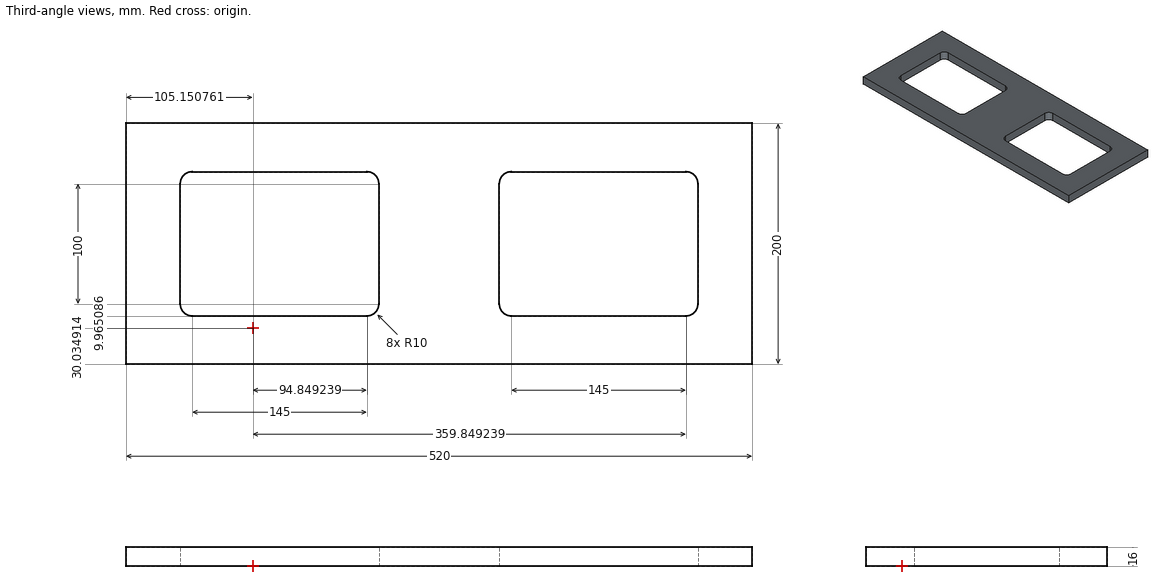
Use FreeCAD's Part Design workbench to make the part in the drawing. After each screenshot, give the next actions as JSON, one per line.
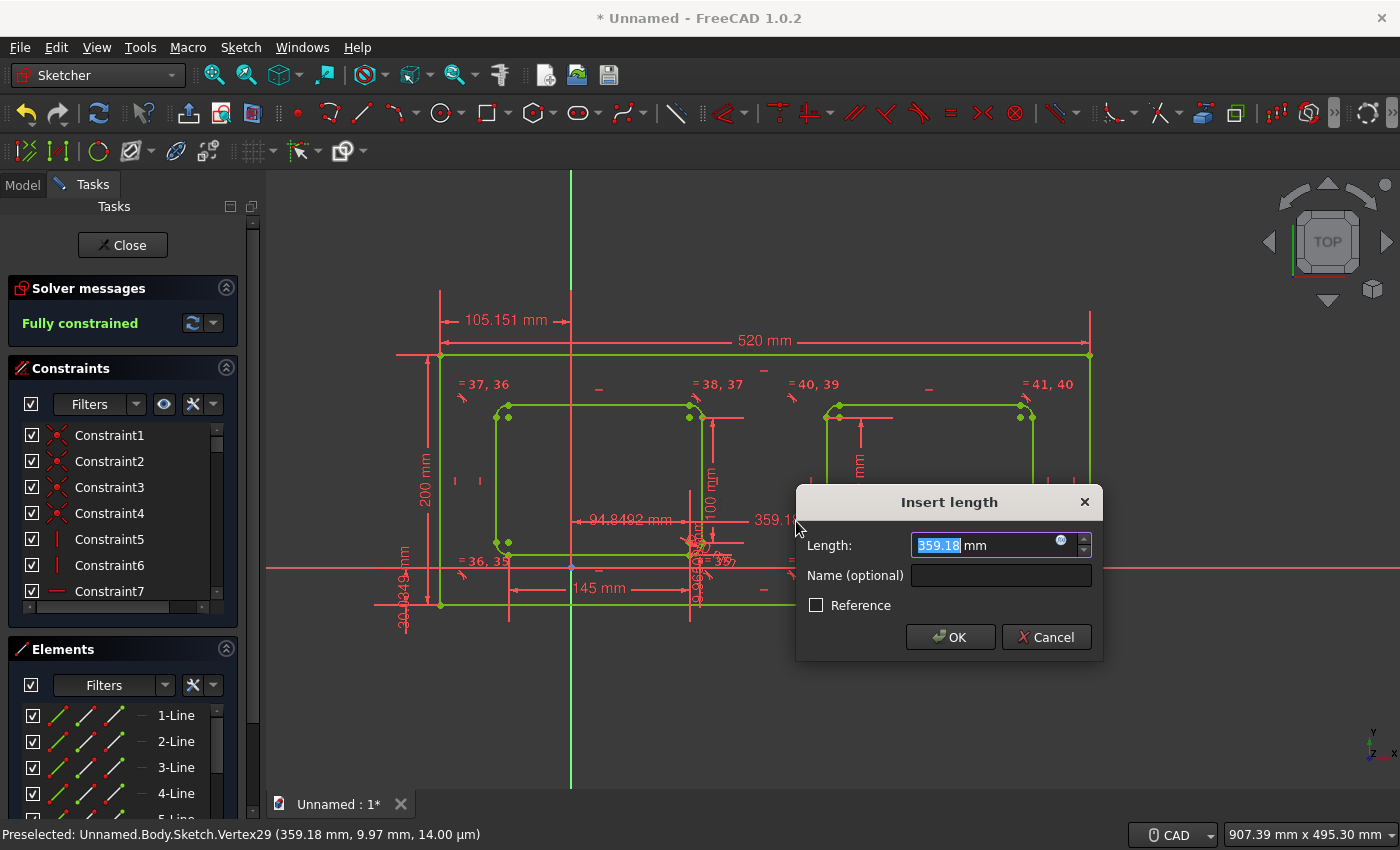
{"action": "type", "text": "359.849239"}
{"action": "key", "text": "Return"}
{"action": "key", "text": "Escape"}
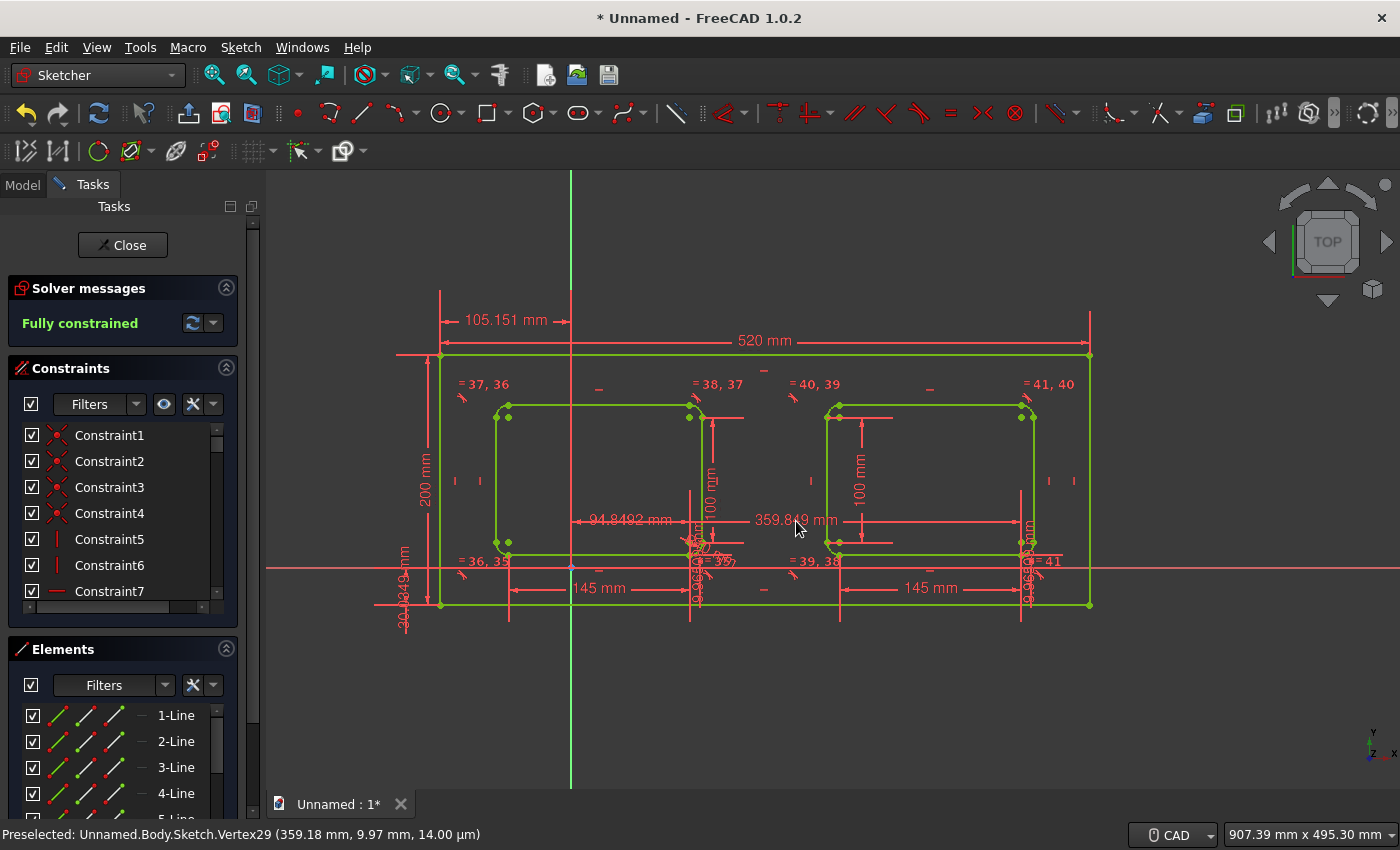
{"action": "left_click", "coordinate": [123, 245]}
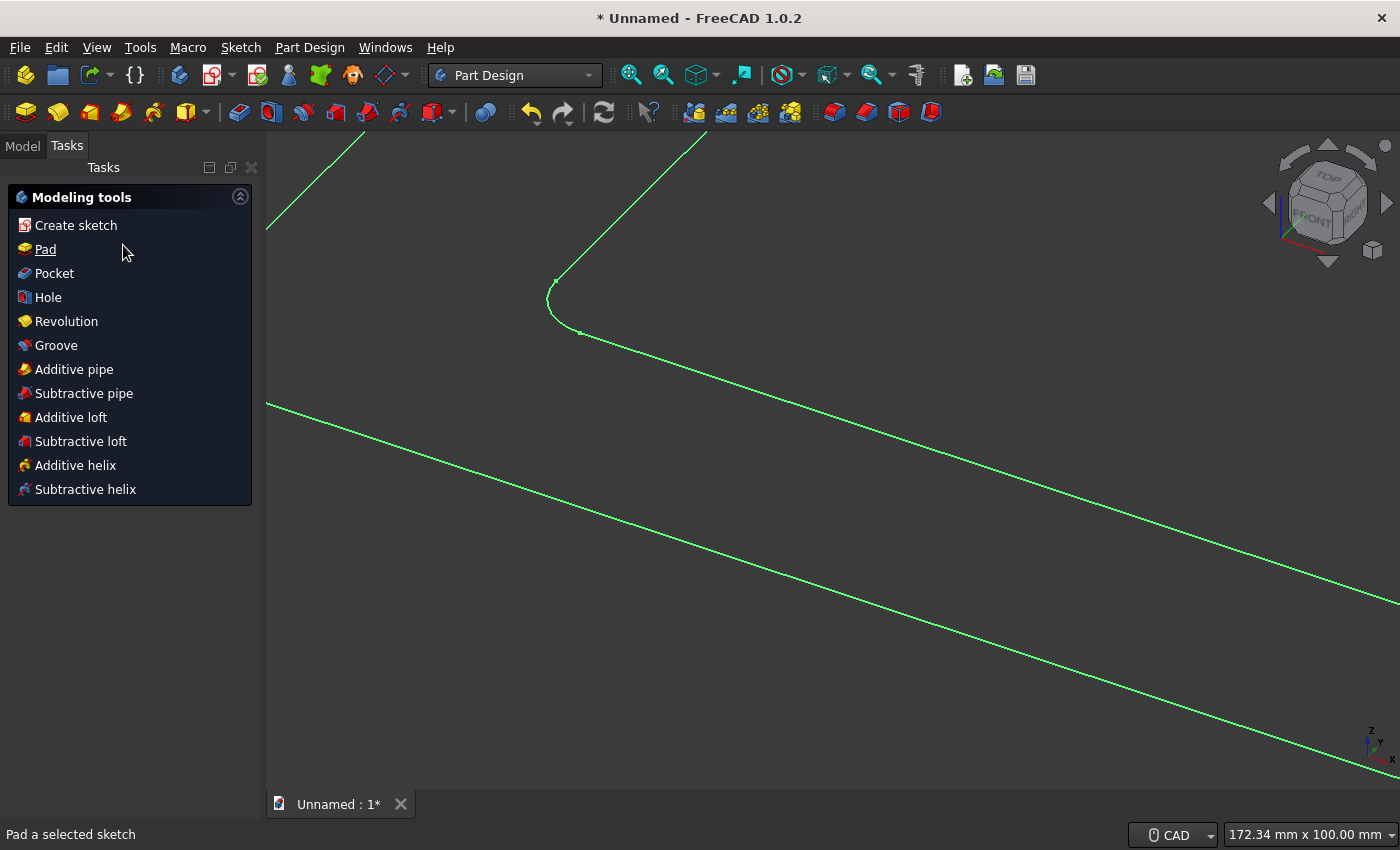
{"action": "left_click", "coordinate": [26, 112]}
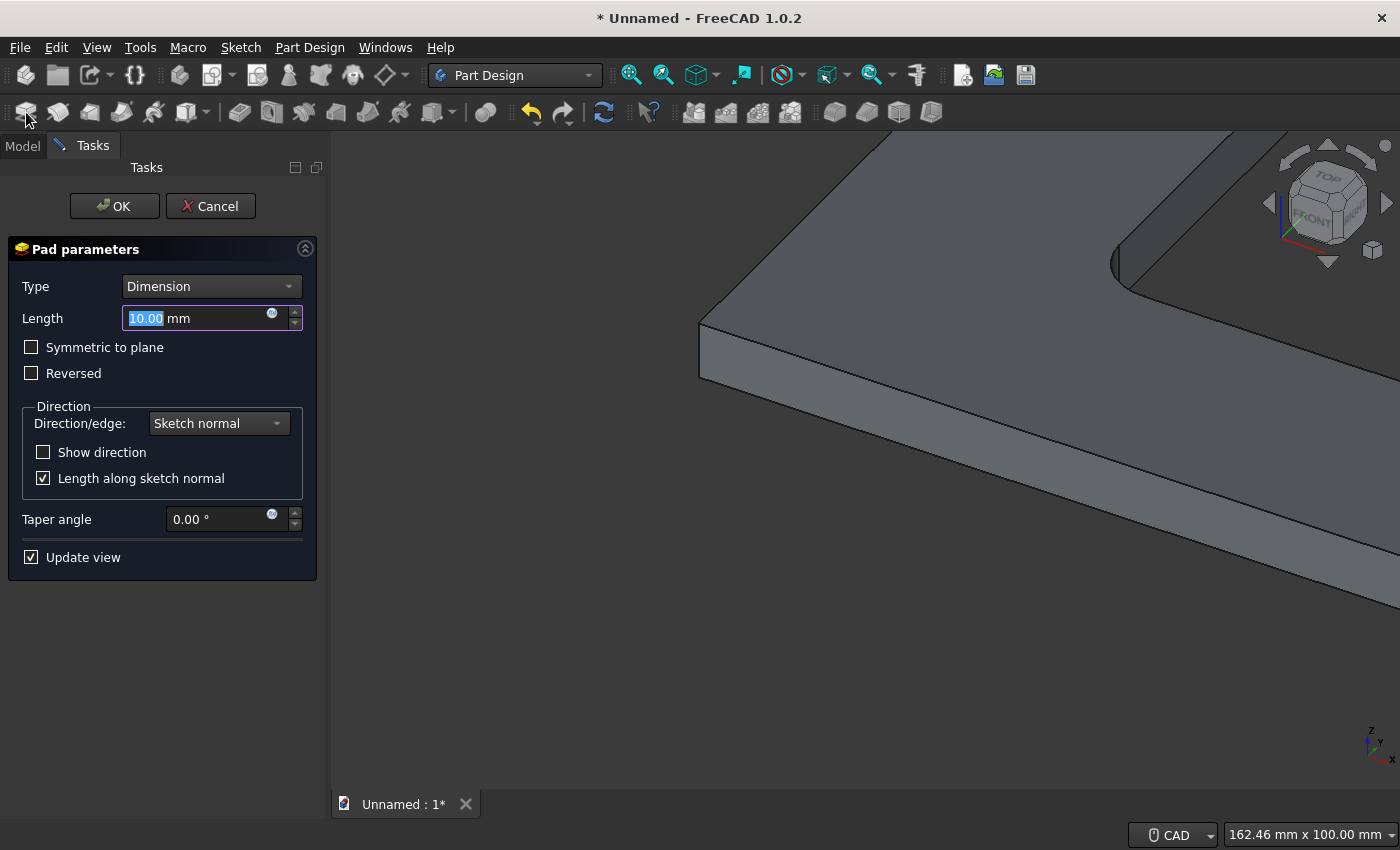
{"action": "type", "text": "16"}
{"action": "key", "text": "Tab"}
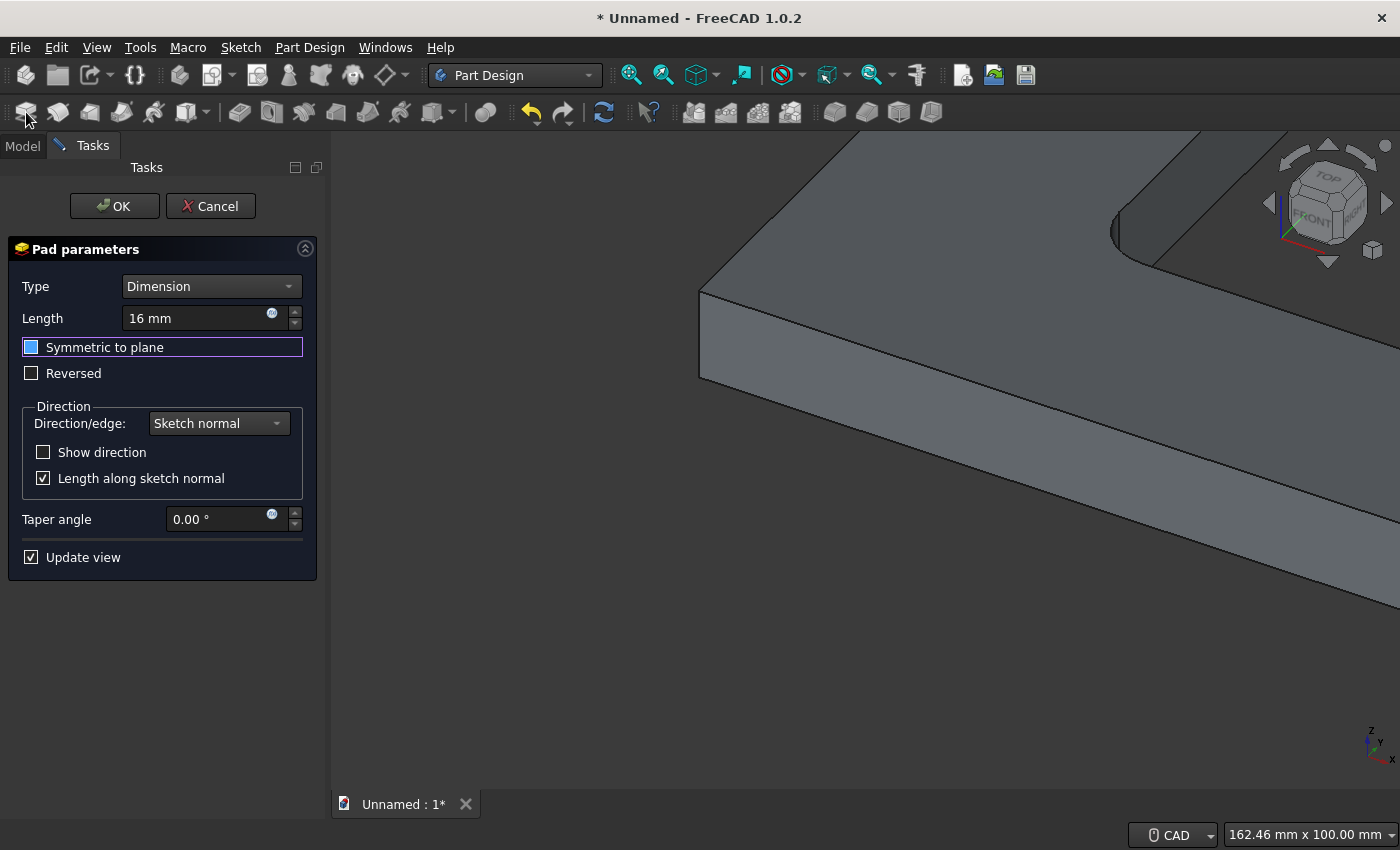
{"action": "left_click", "coordinate": [115, 206]}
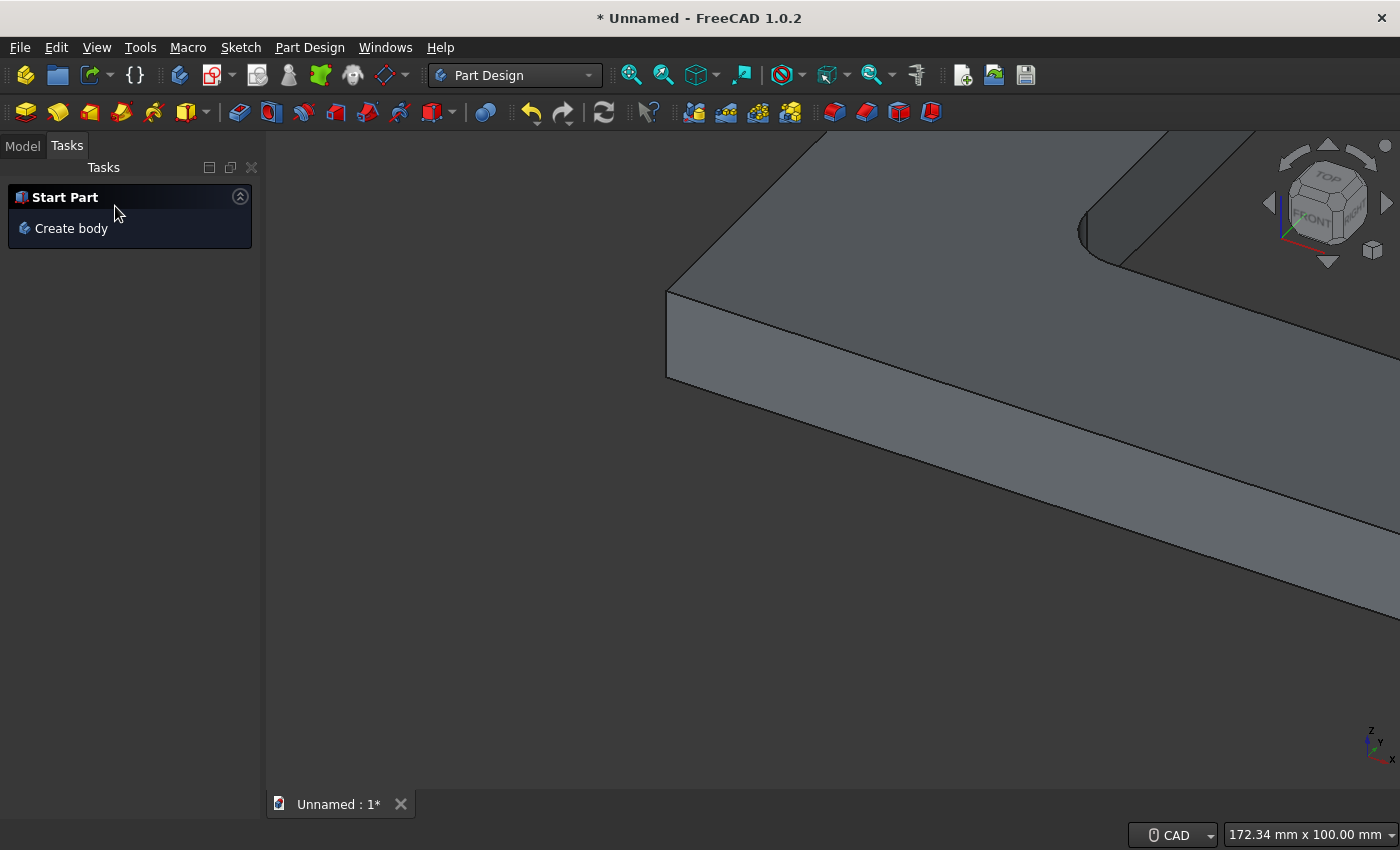
{"action": "key", "text": "0"}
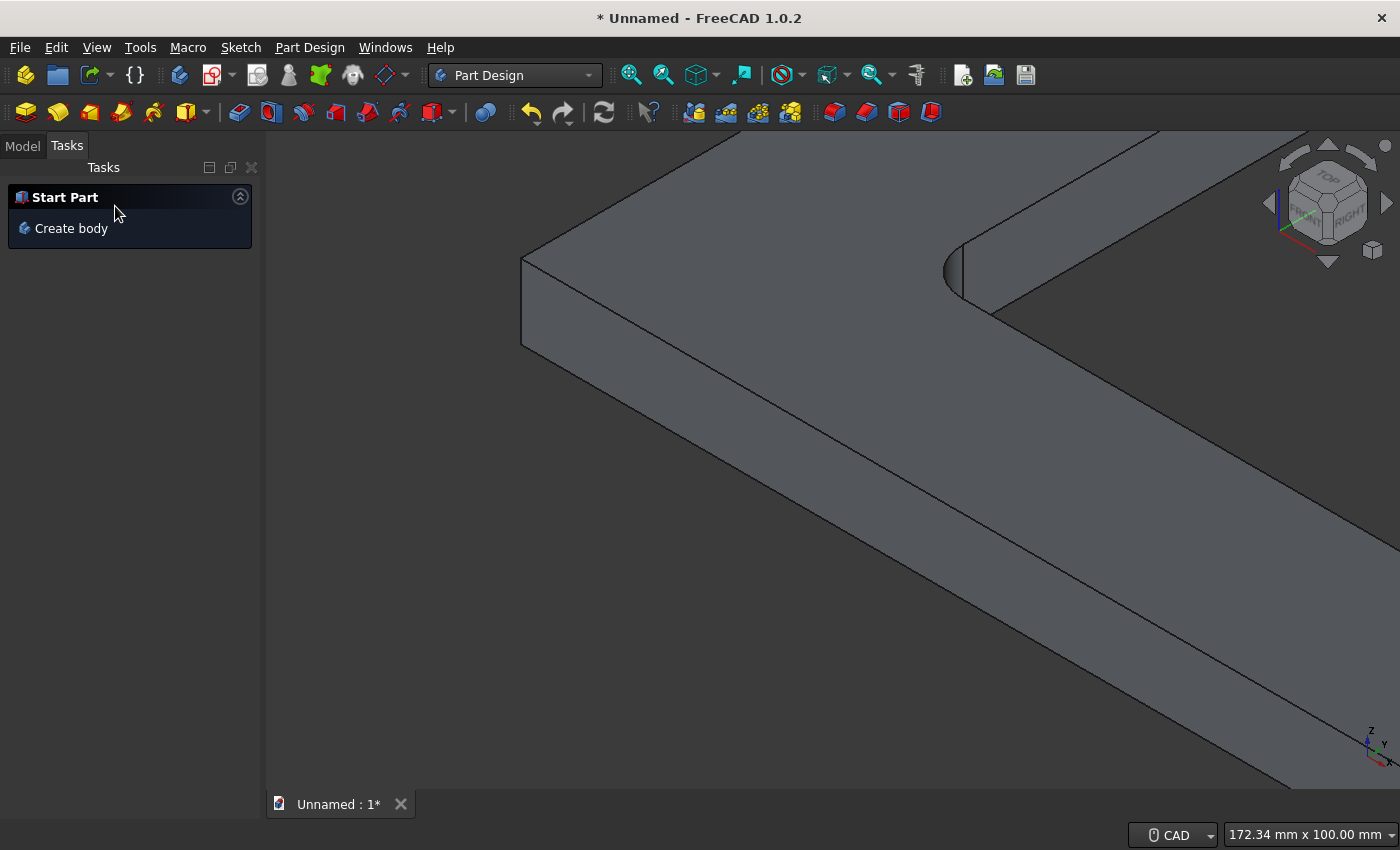
{"action": "key", "text": "v f"}